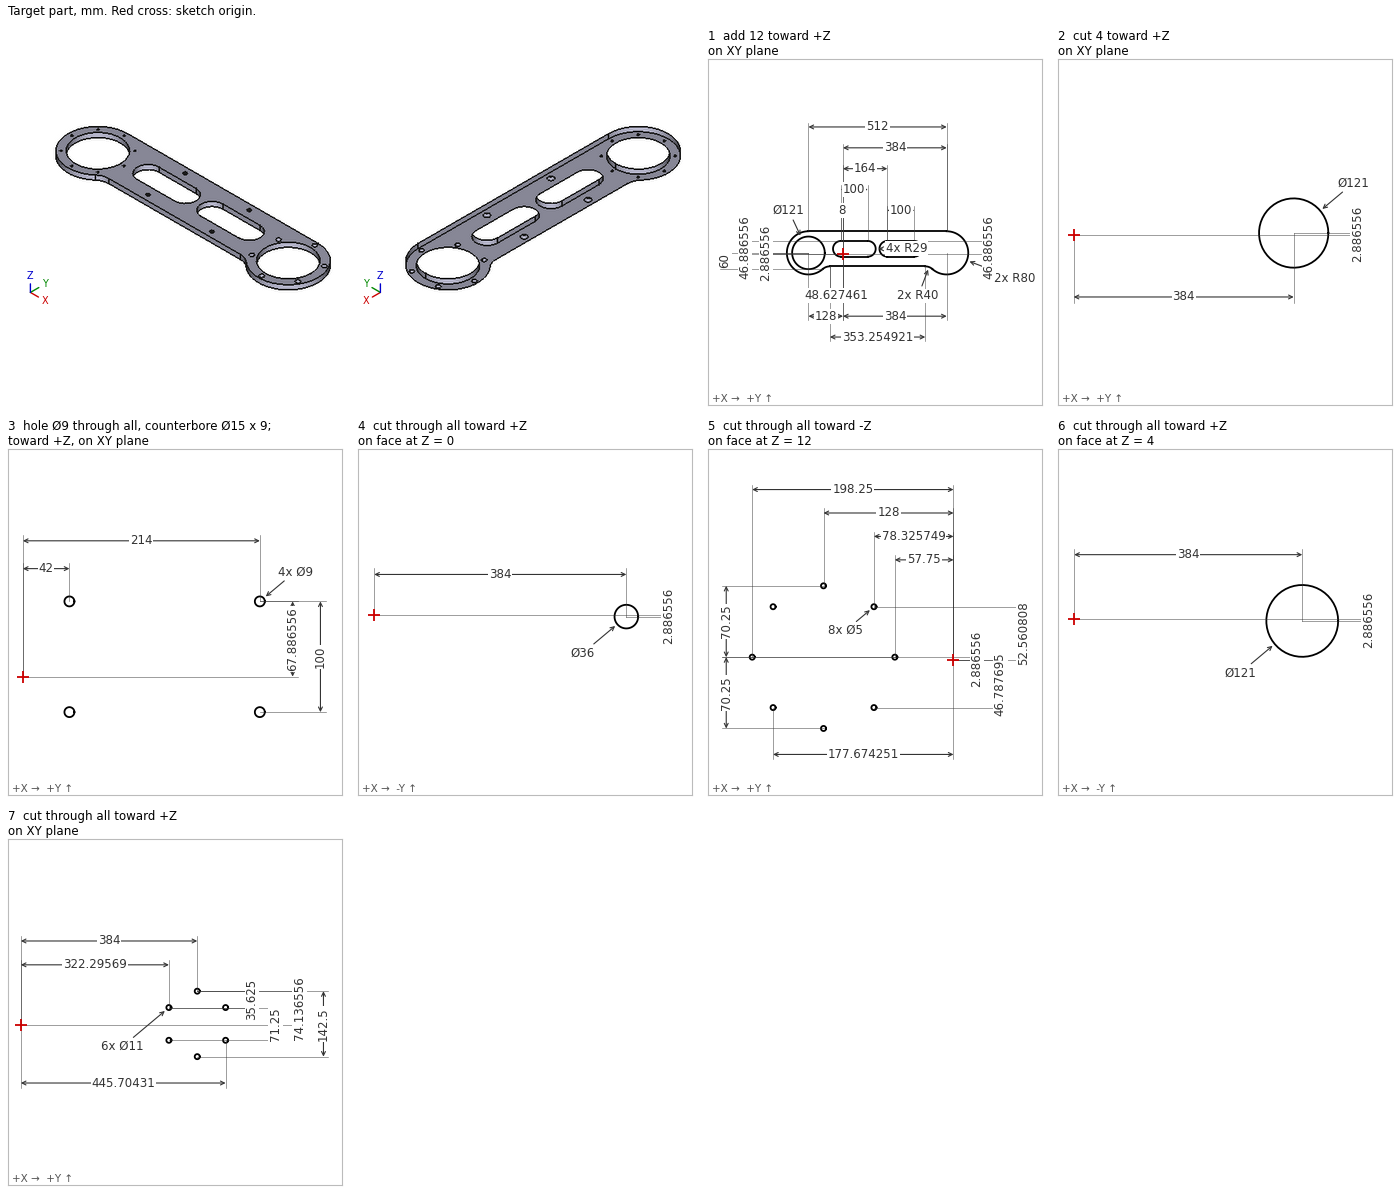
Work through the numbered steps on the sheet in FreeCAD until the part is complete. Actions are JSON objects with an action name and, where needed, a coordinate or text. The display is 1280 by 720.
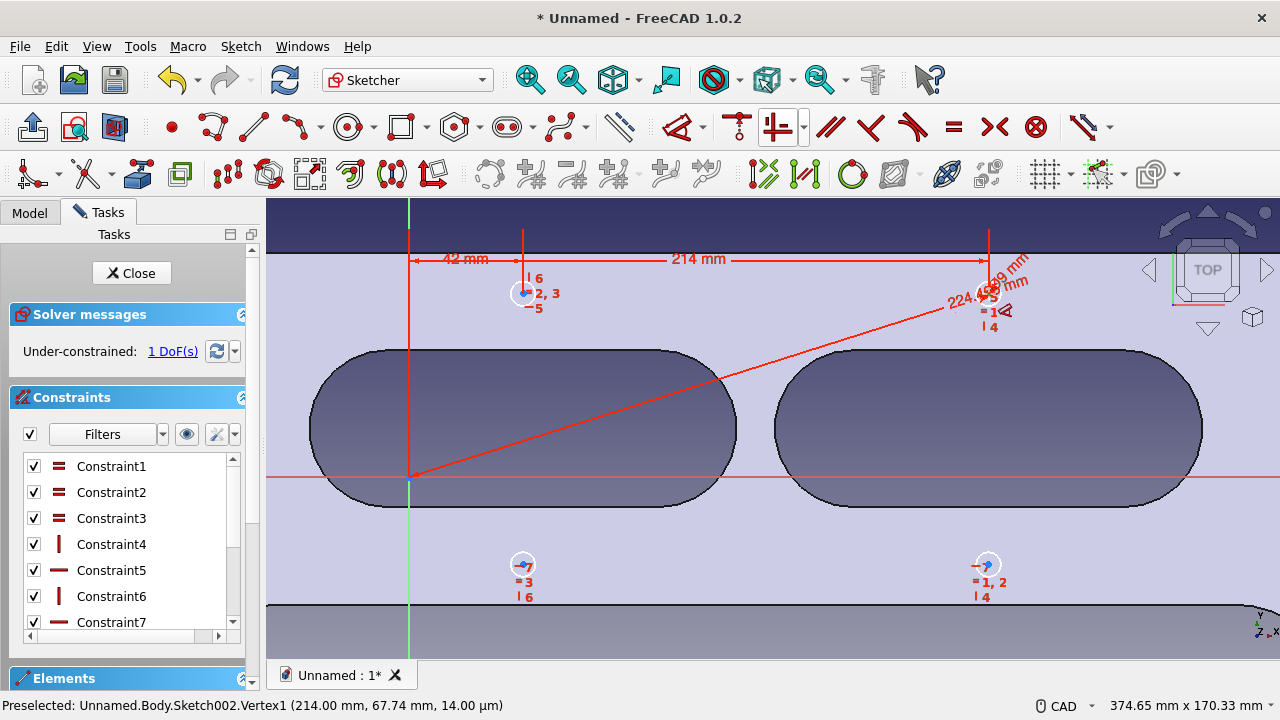
{"action": "left_click", "coordinate": [989, 565]}
{"action": "left_click", "coordinate": [1023, 429]}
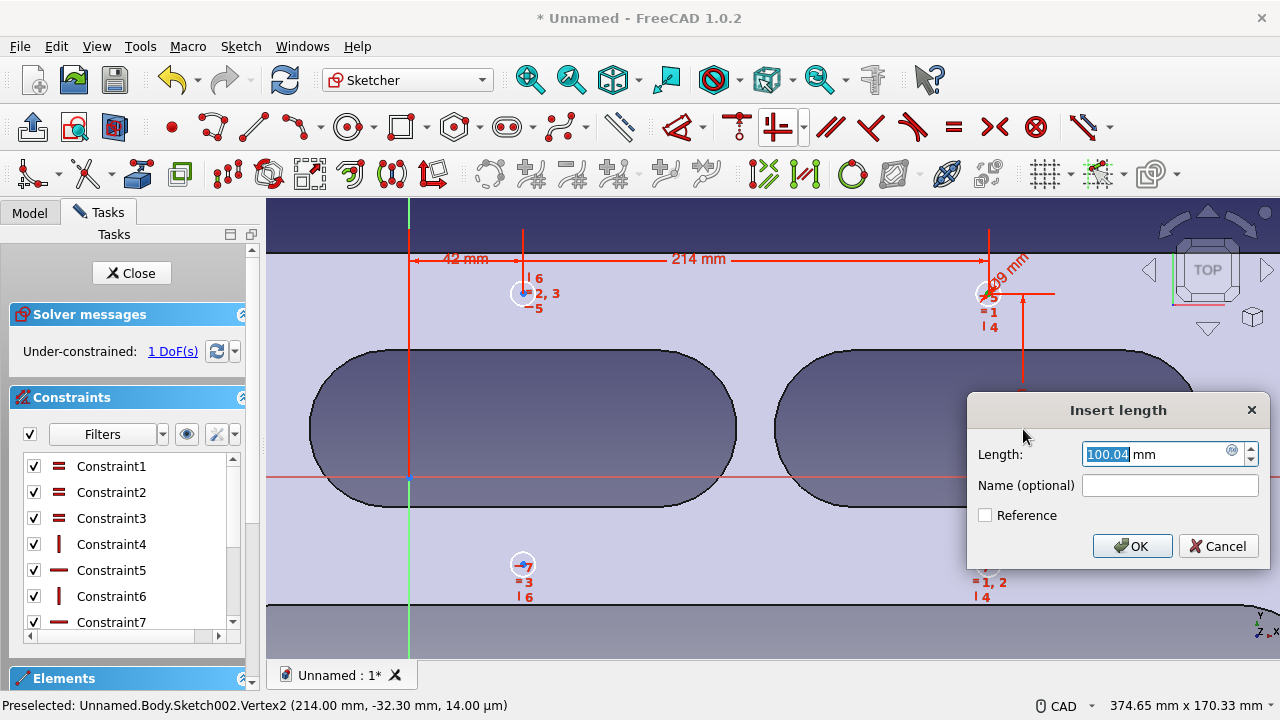
{"action": "type", "text": "100"}
{"action": "key", "text": "Return"}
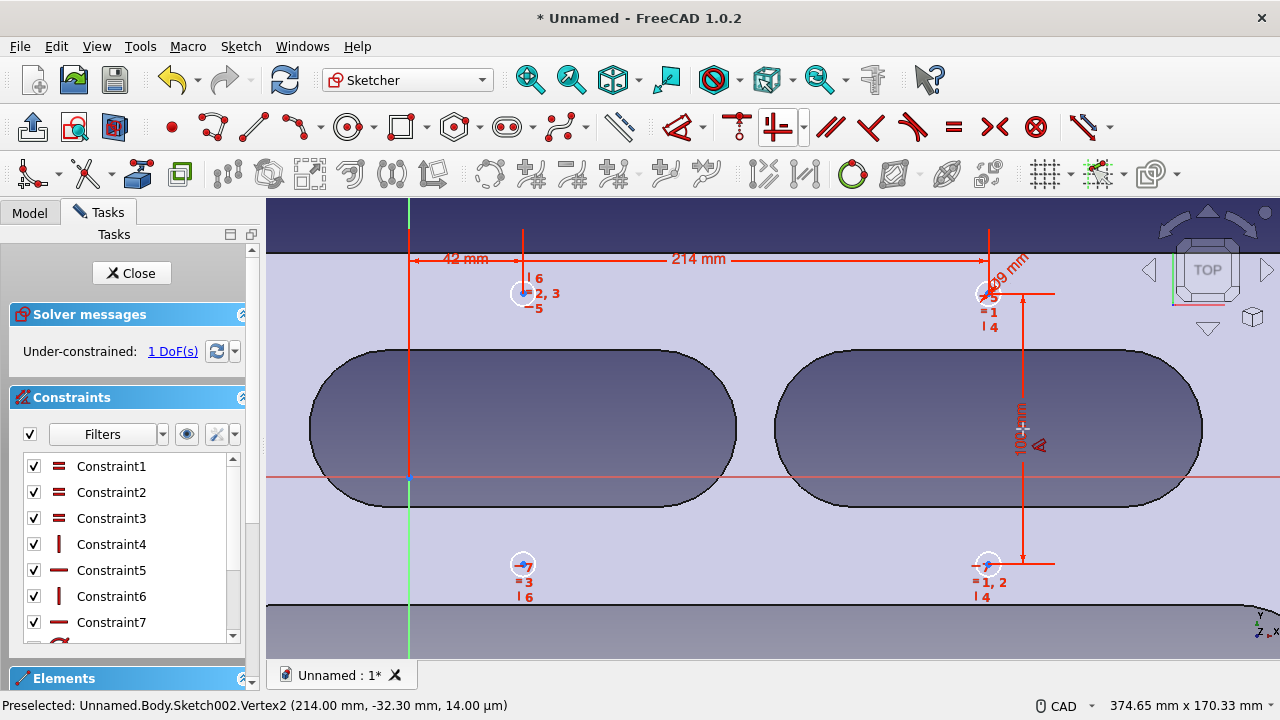
{"action": "left_click", "coordinate": [989, 294]}
{"action": "left_click", "coordinate": [375, 385]}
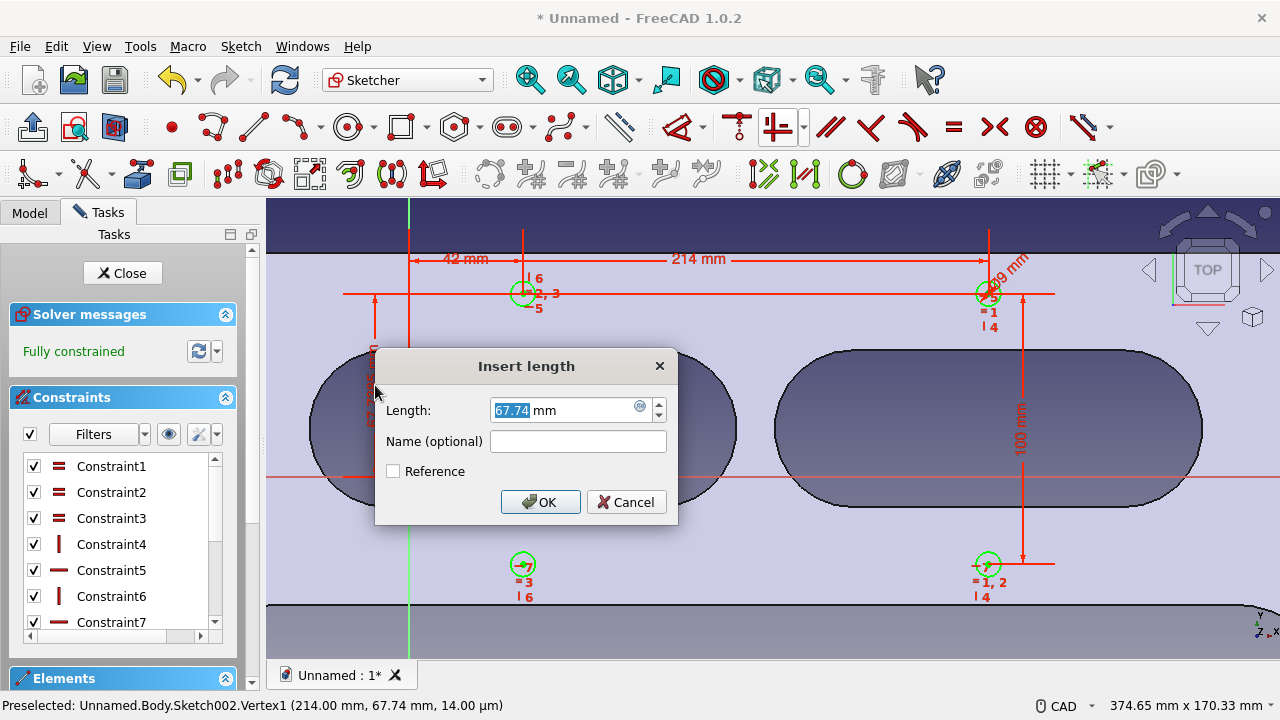
{"action": "type", "text": "67.886556"}
{"action": "key", "text": "Return"}
{"action": "key", "text": "Escape"}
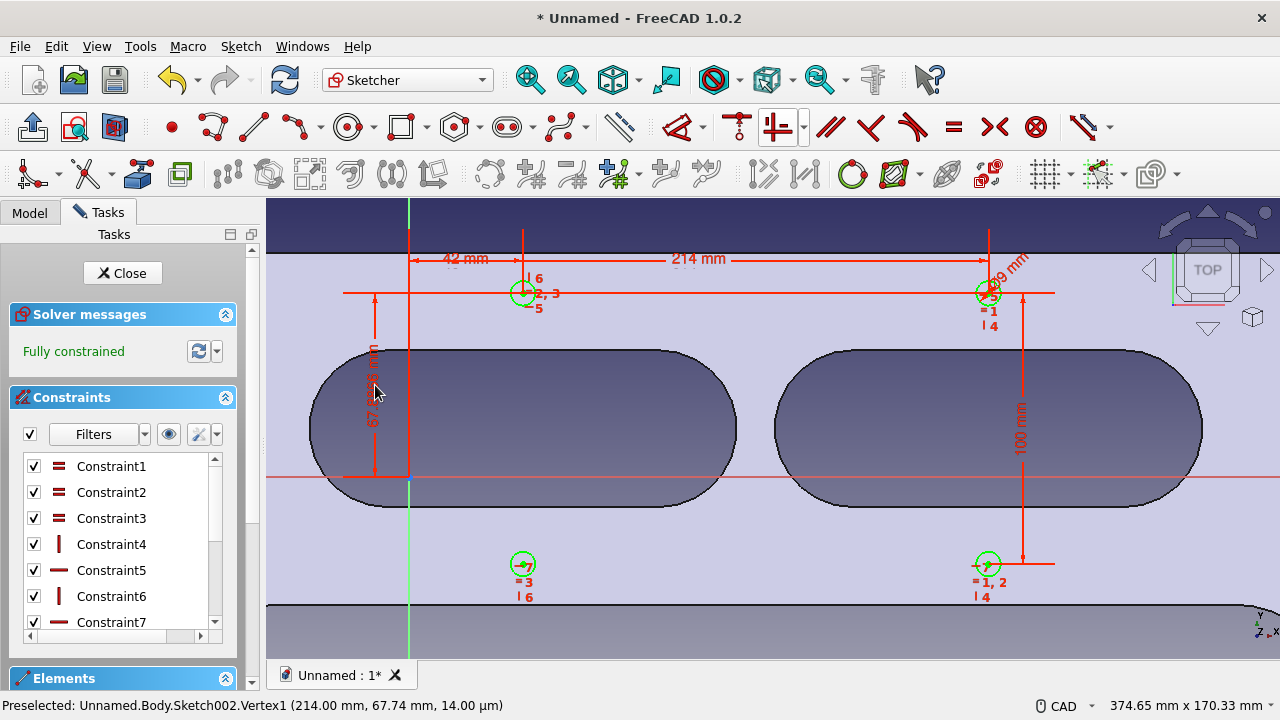
{"action": "left_click", "coordinate": [123, 273]}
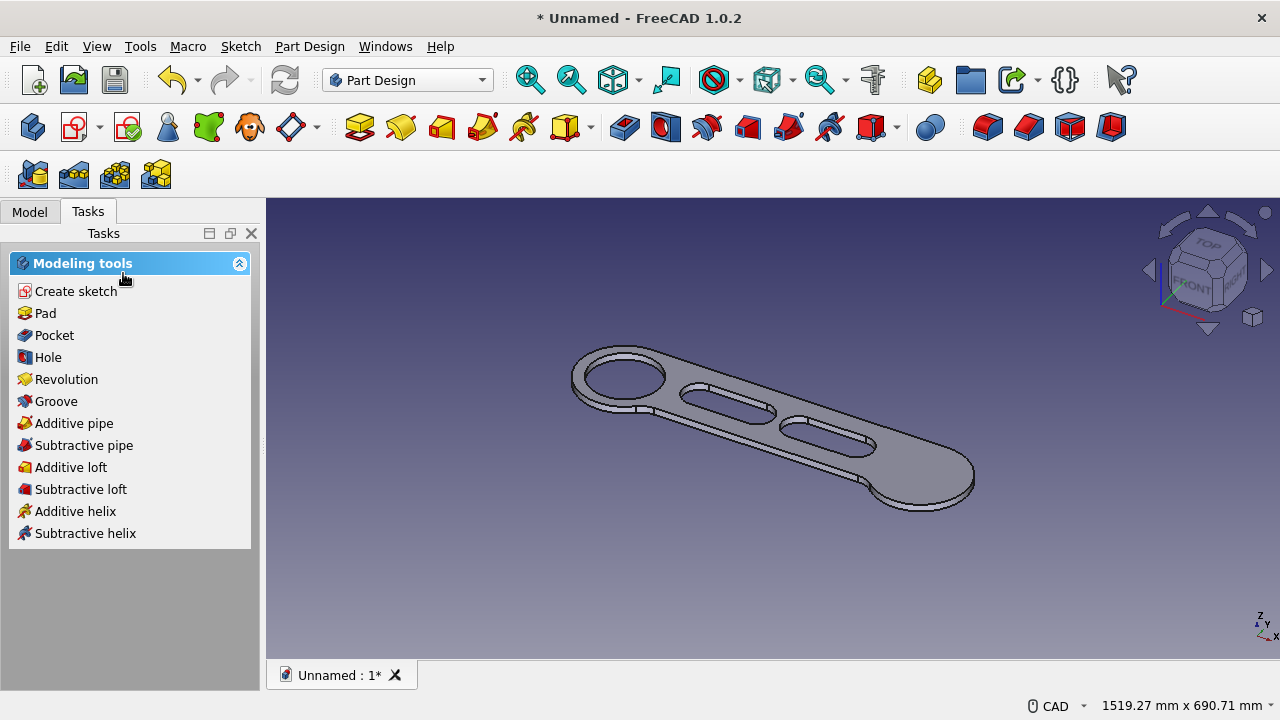
{"action": "left_click", "coordinate": [666, 128]}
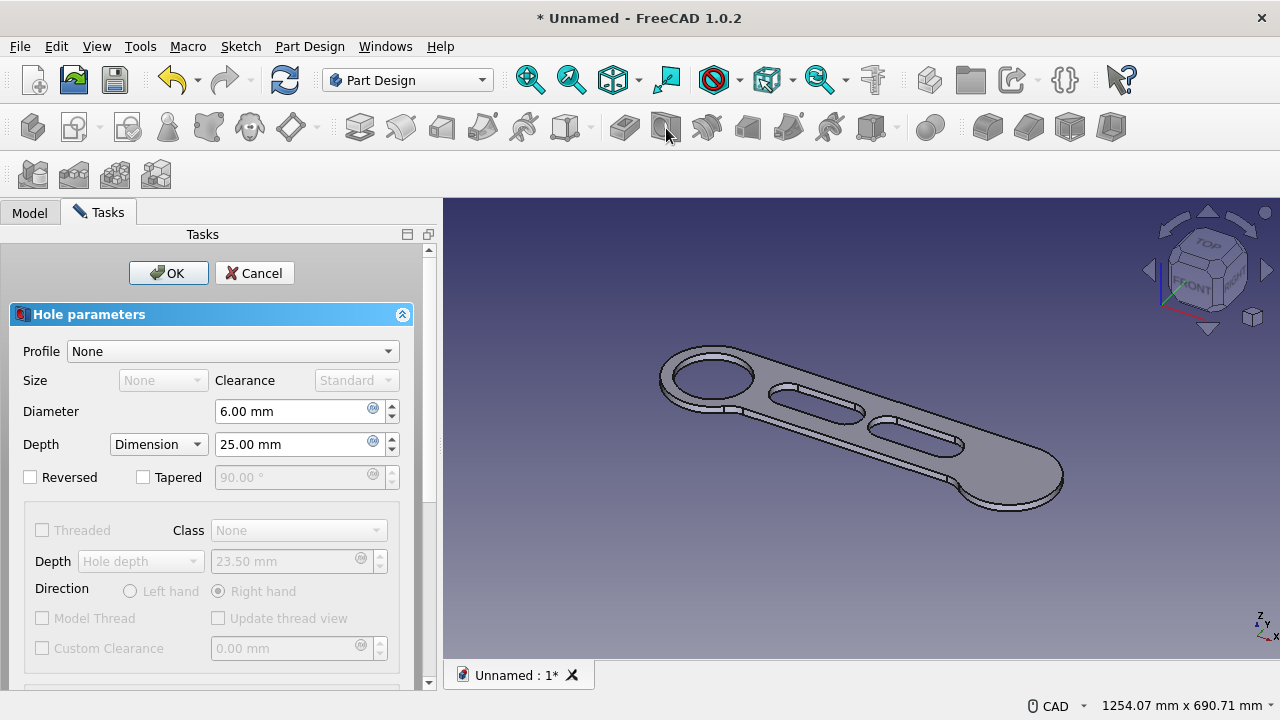
{"action": "triple_click", "coordinate": [300, 412]}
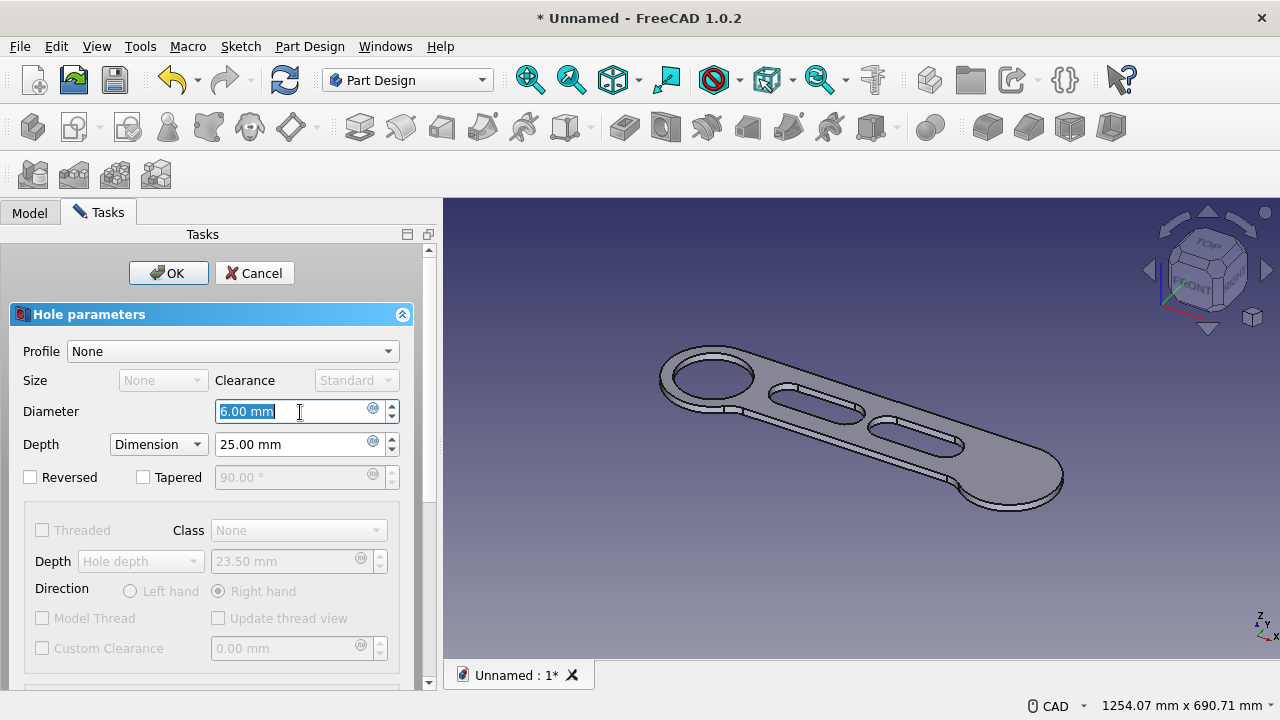
{"action": "type", "text": "9"}
{"action": "key", "text": "Tab"}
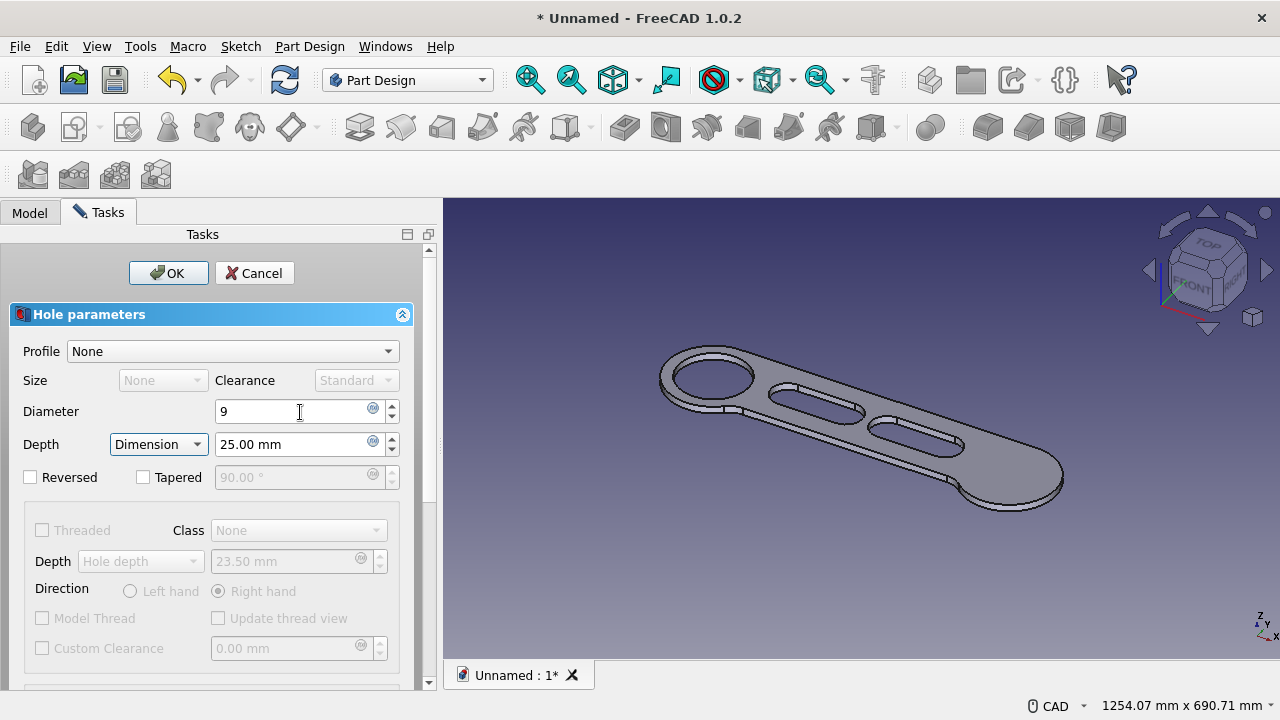
{"action": "left_click", "coordinate": [160, 444]}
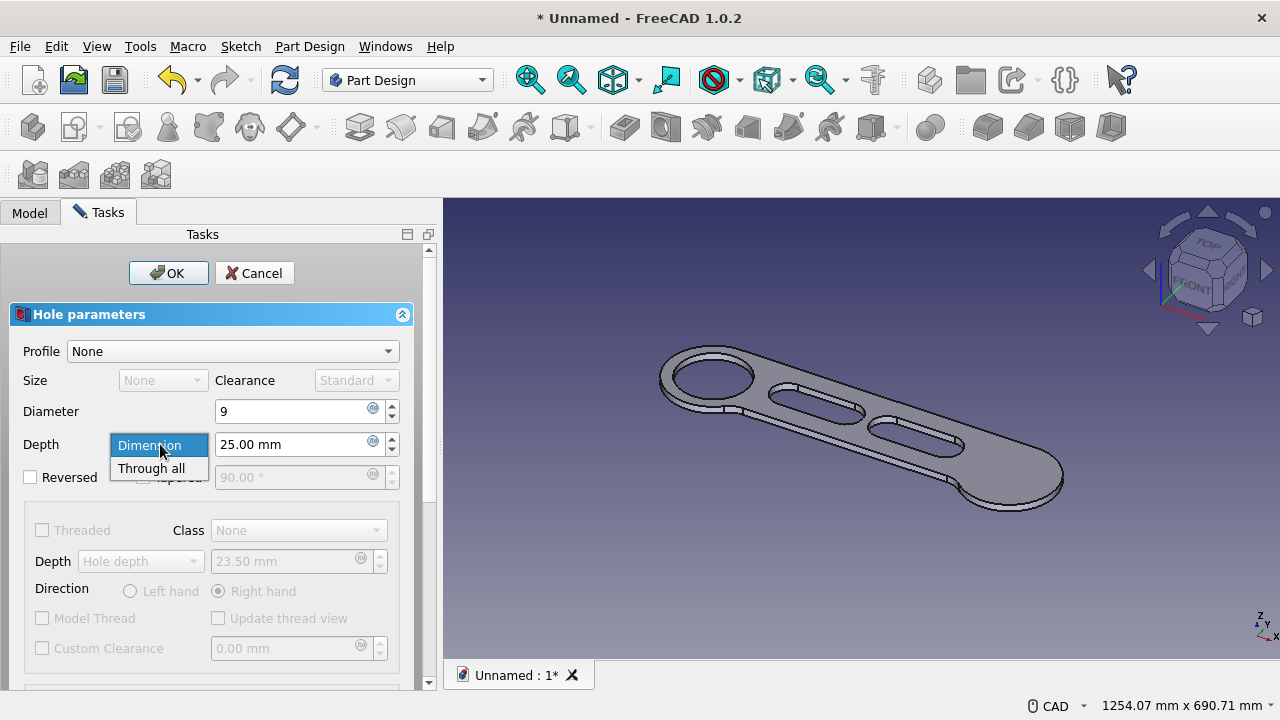
{"action": "left_click", "coordinate": [158, 468]}